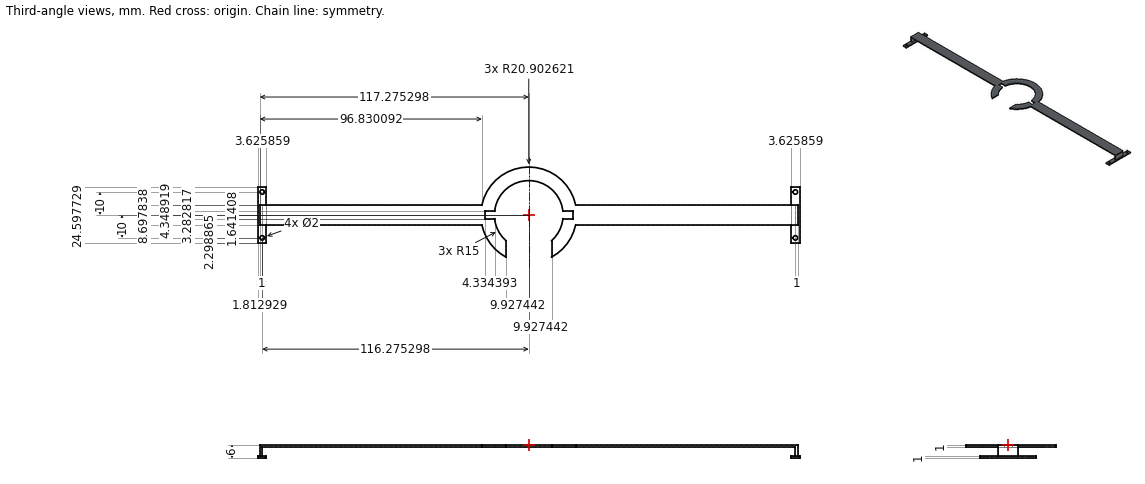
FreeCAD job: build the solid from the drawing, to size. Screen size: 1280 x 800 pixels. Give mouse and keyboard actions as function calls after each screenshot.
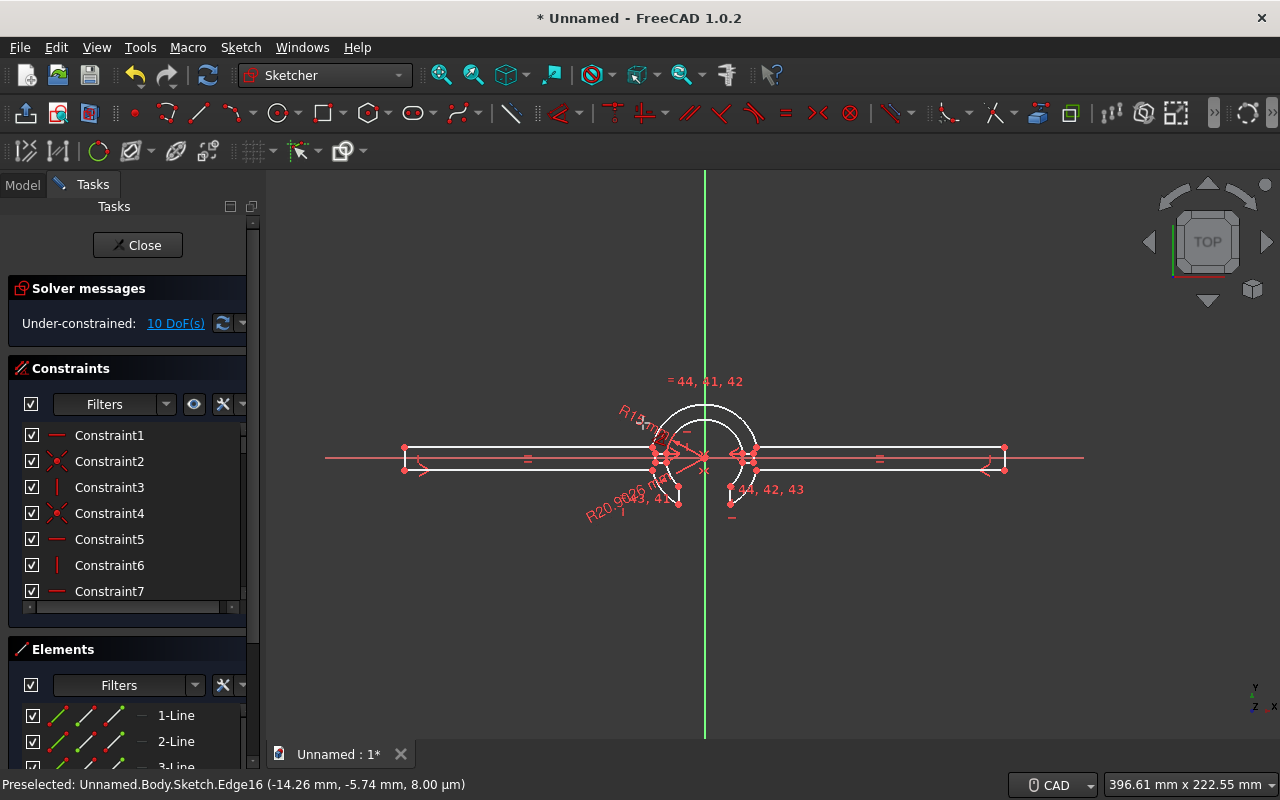
scroll(405, 457, up, 3)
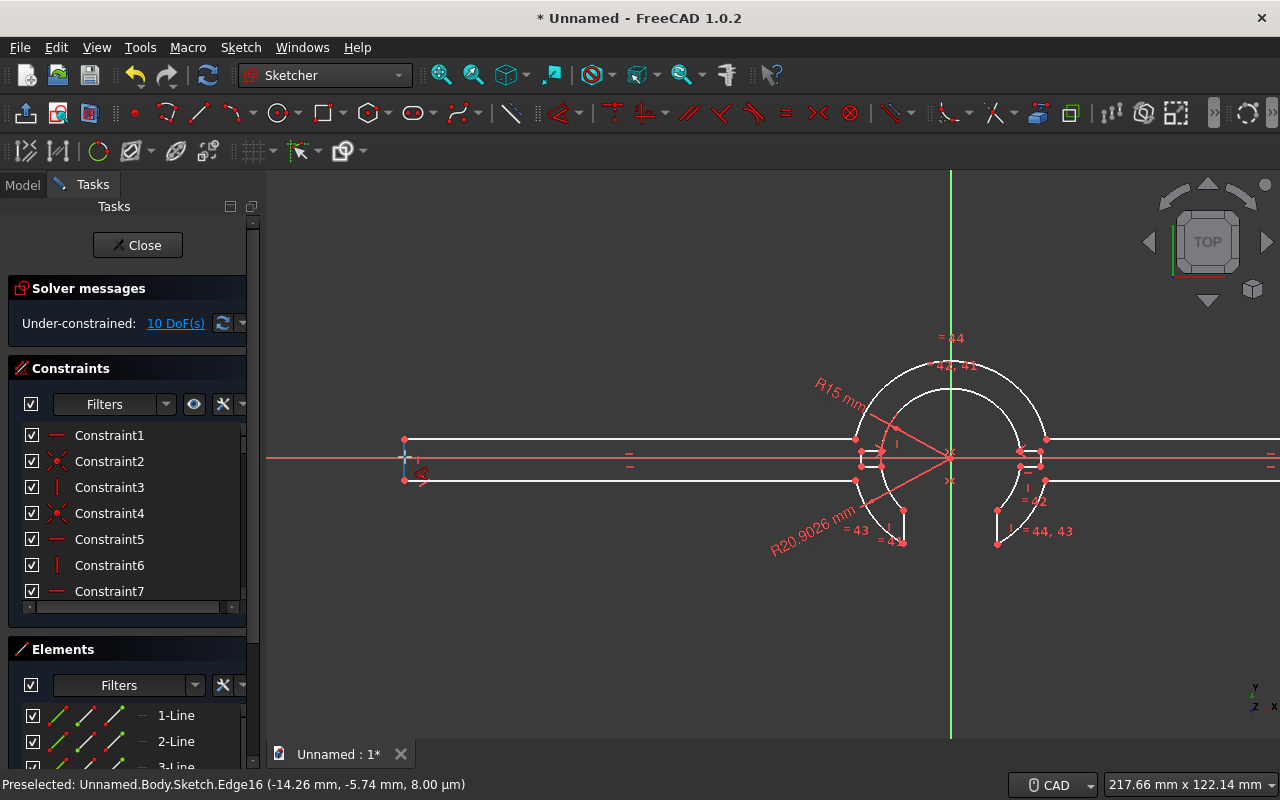
click(404, 456)
click(370, 445)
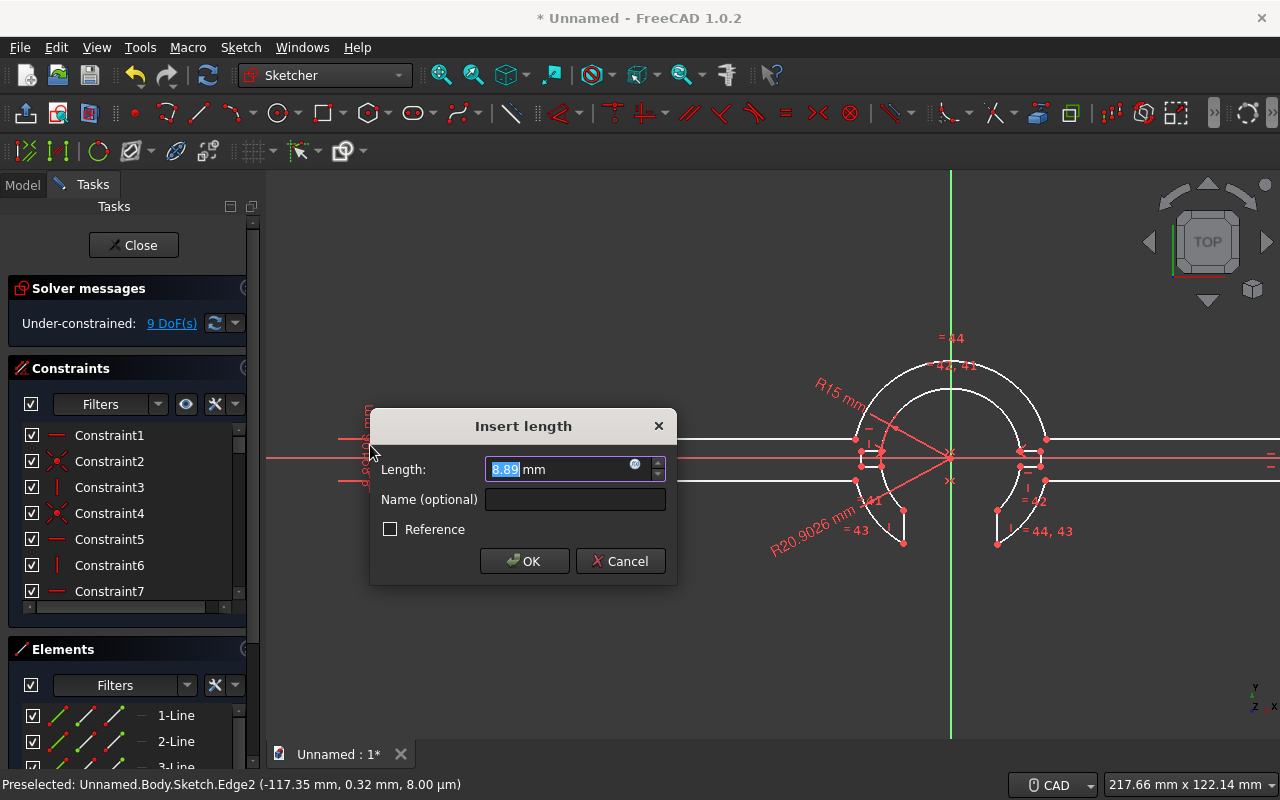
text(8.697838)
key(Return)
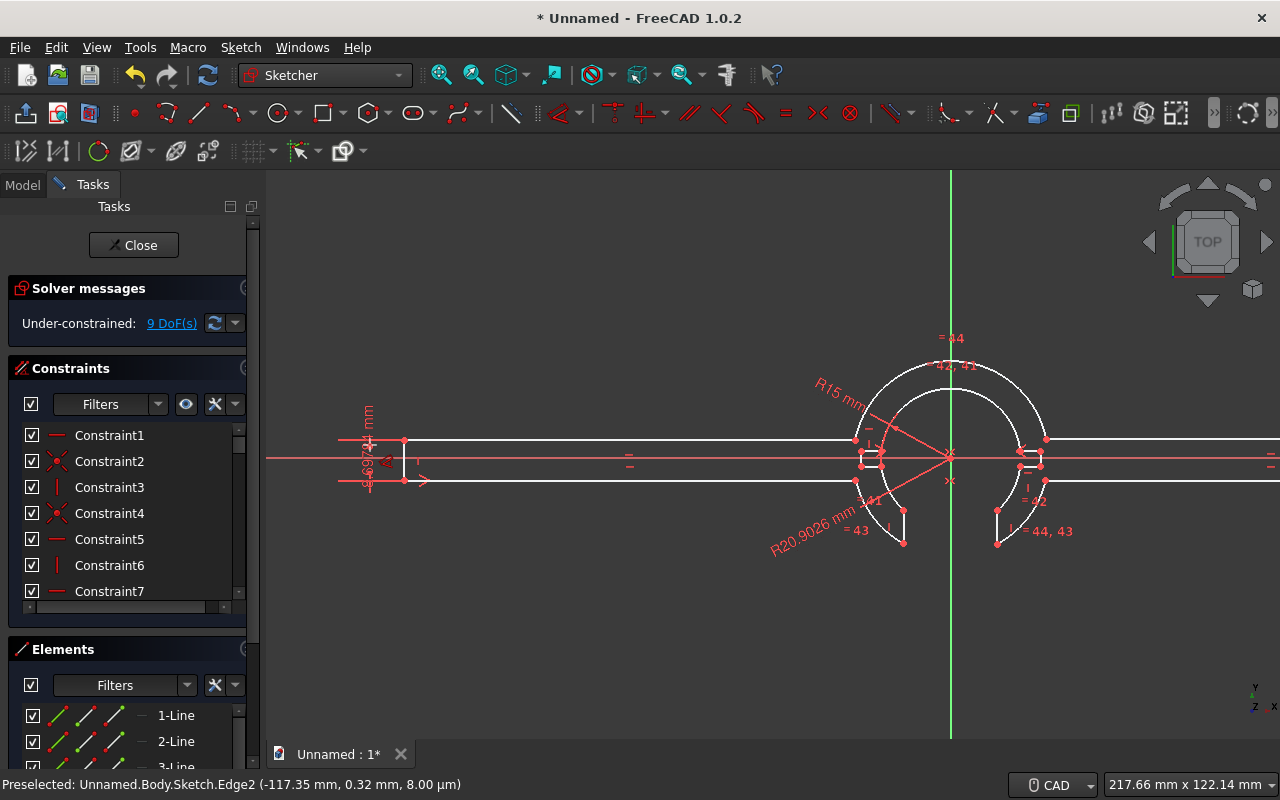
scroll(871, 467, up, 4)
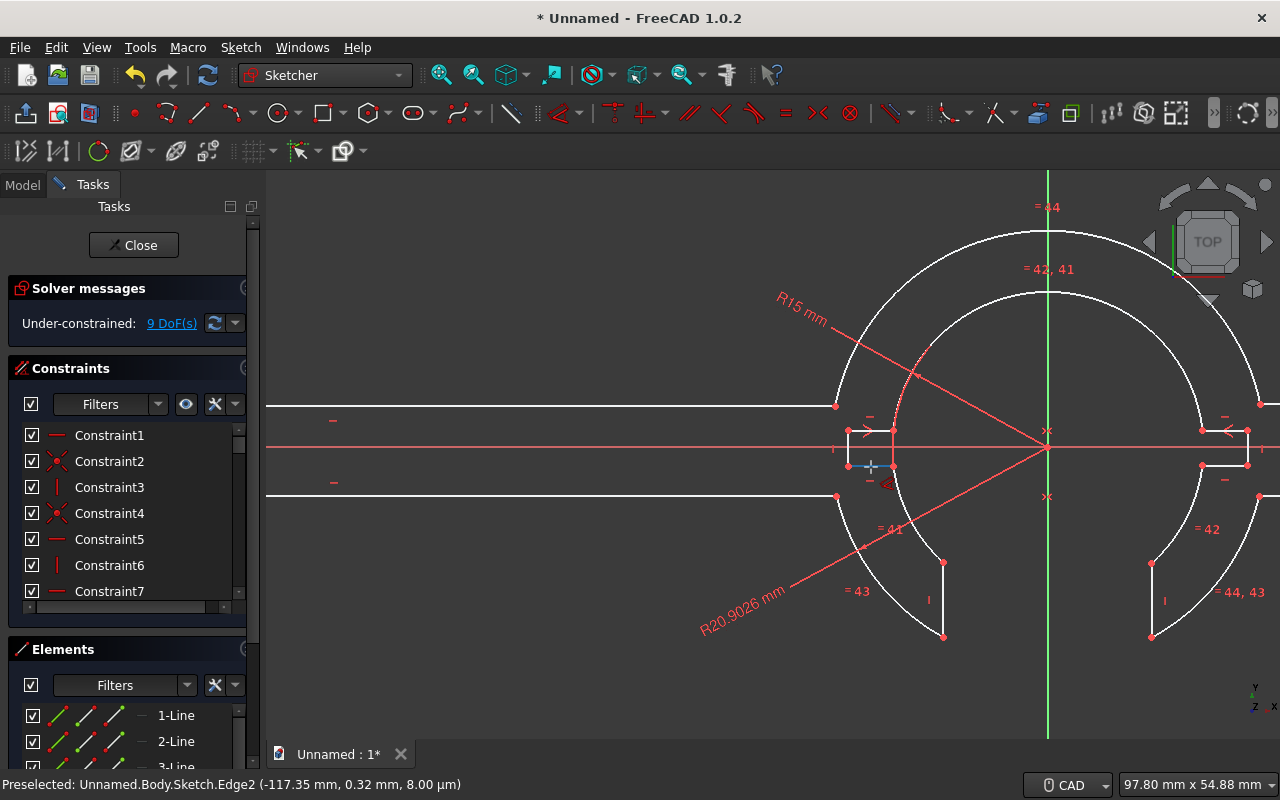
click(871, 466)
click(871, 500)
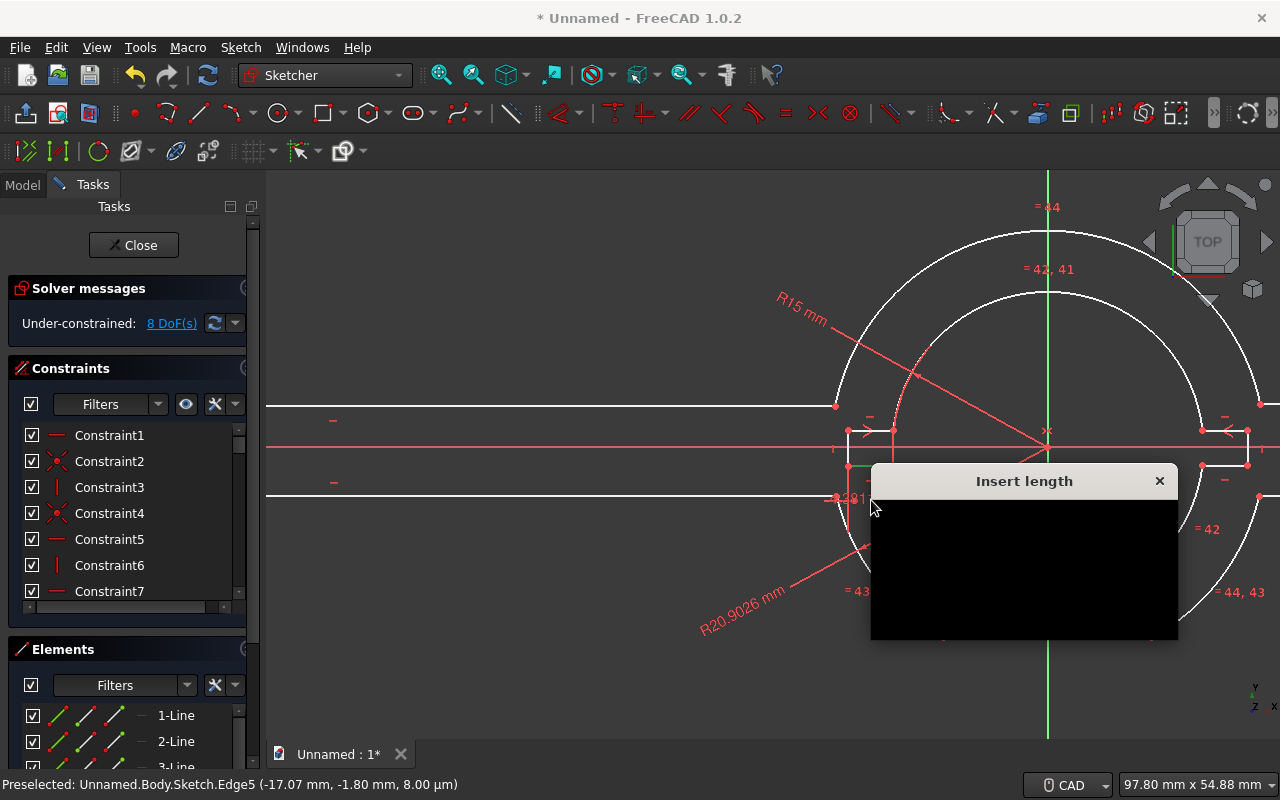
text(4.334393)
key(Return)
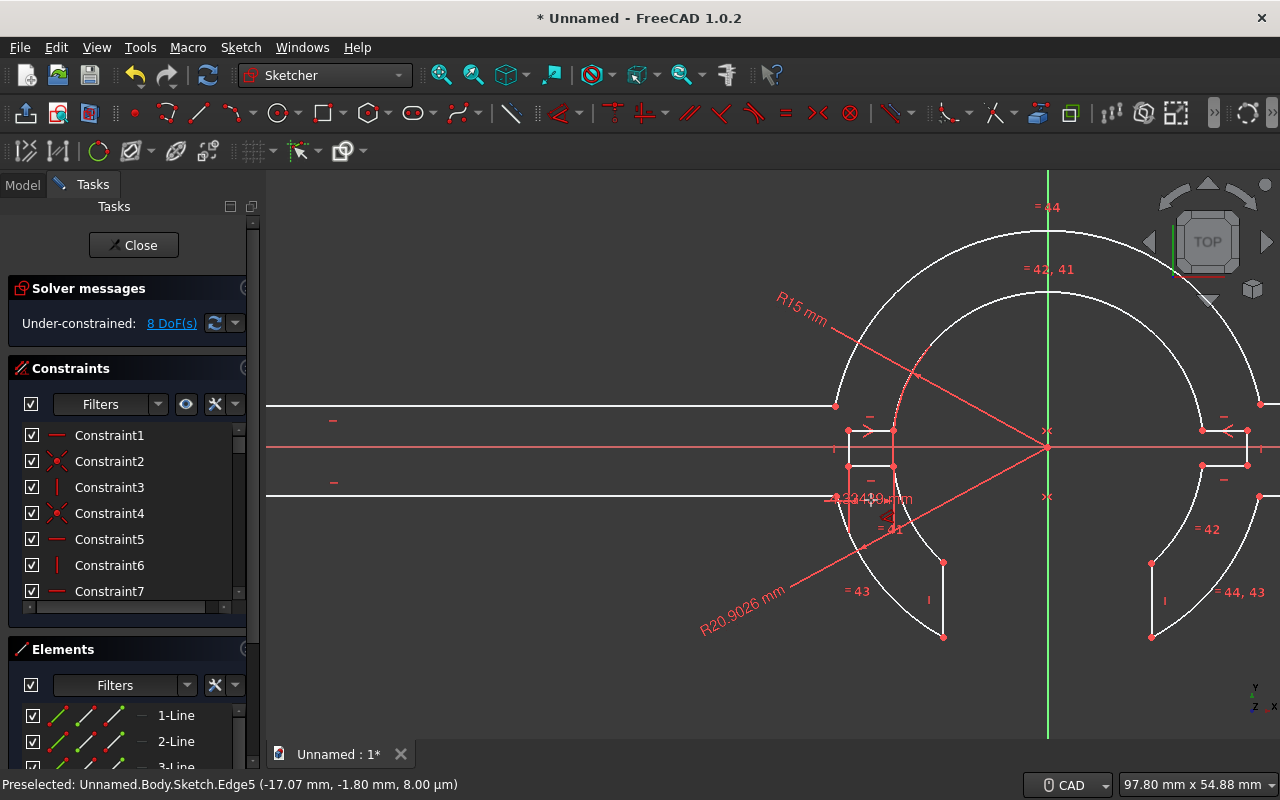
click(849, 445)
click(815, 461)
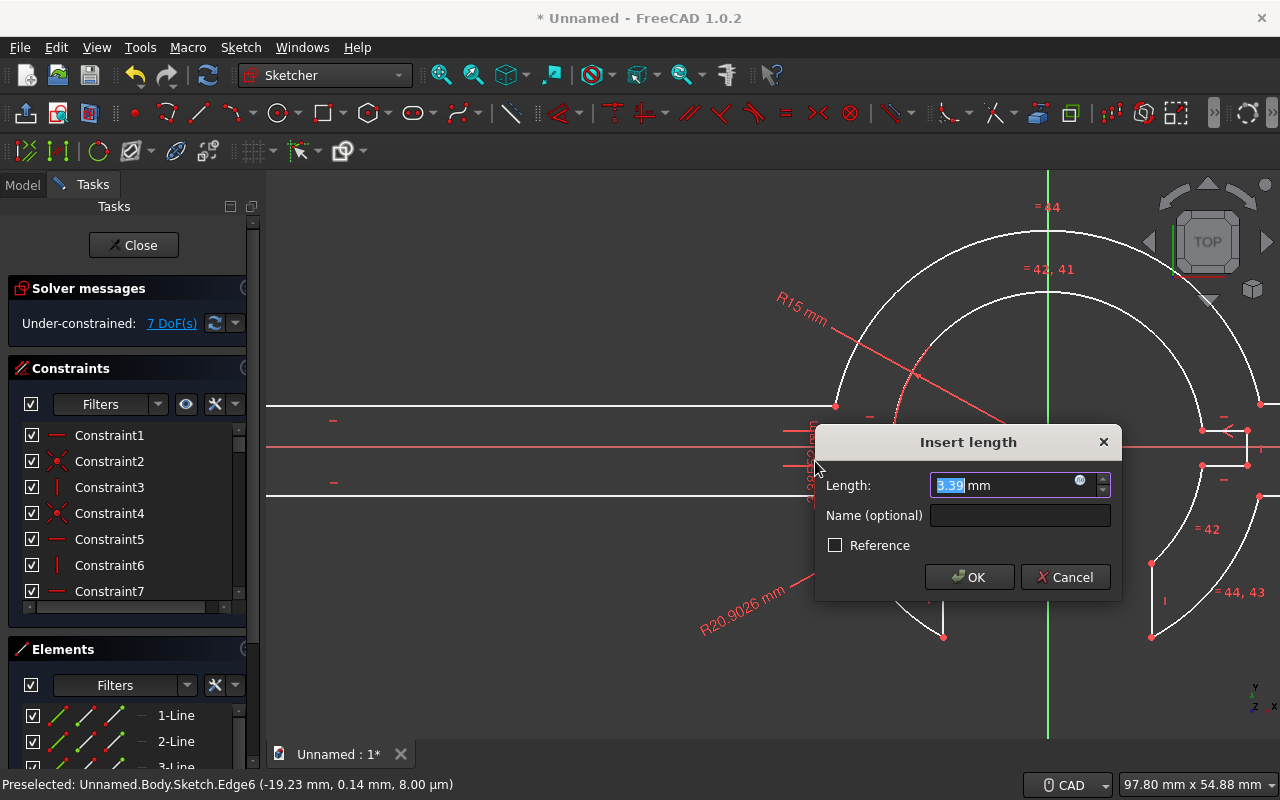
text(3.282817)
key(Return)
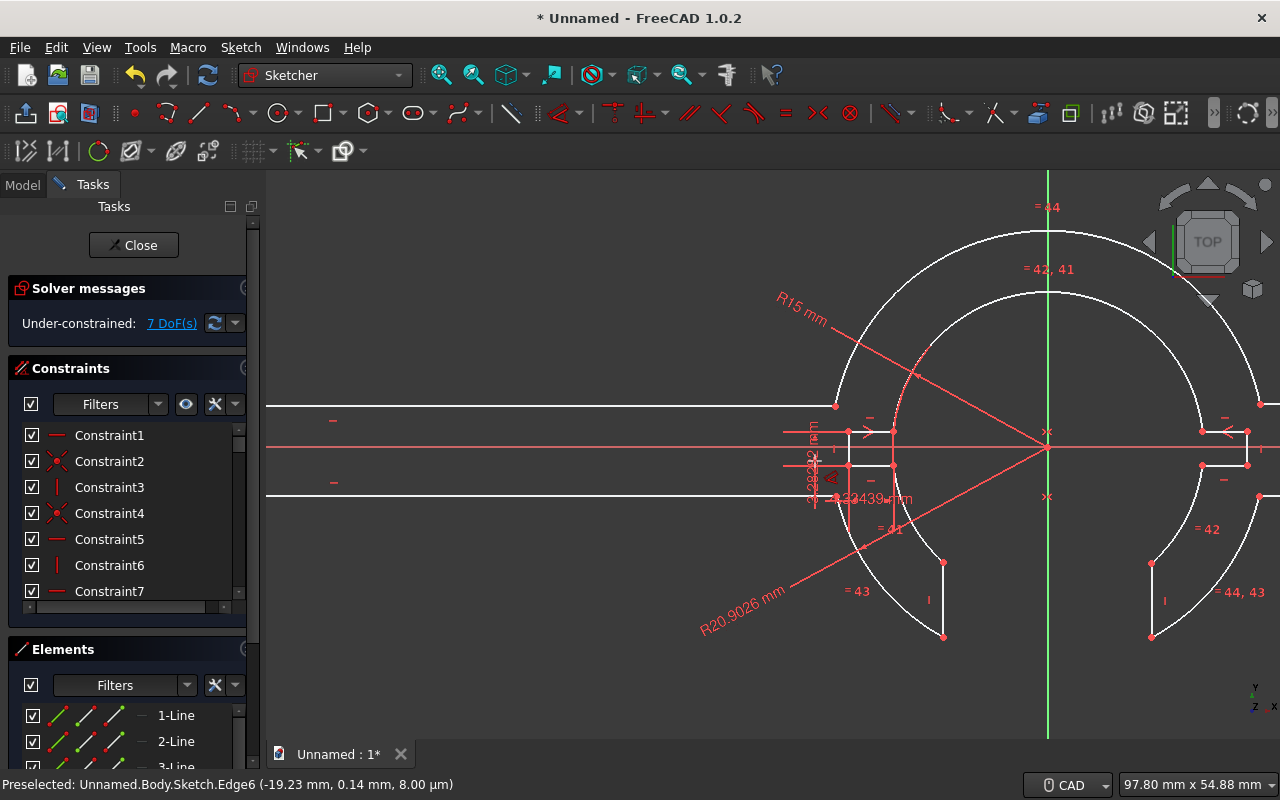
scroll(592, 461, down, 7)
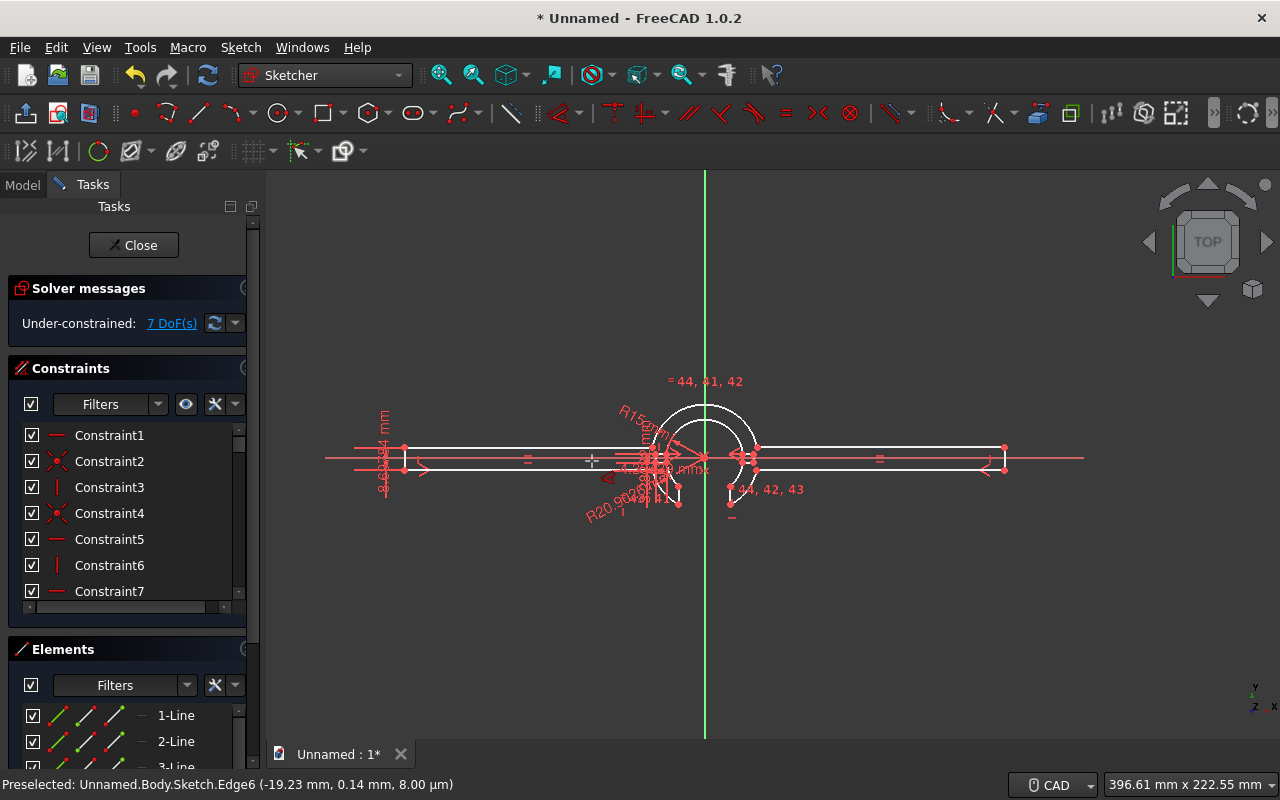
scroll(754, 458, up, 8)